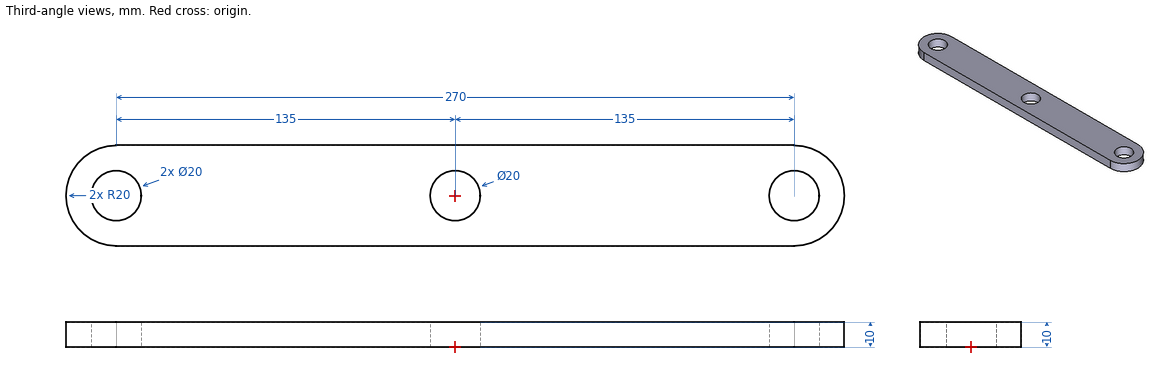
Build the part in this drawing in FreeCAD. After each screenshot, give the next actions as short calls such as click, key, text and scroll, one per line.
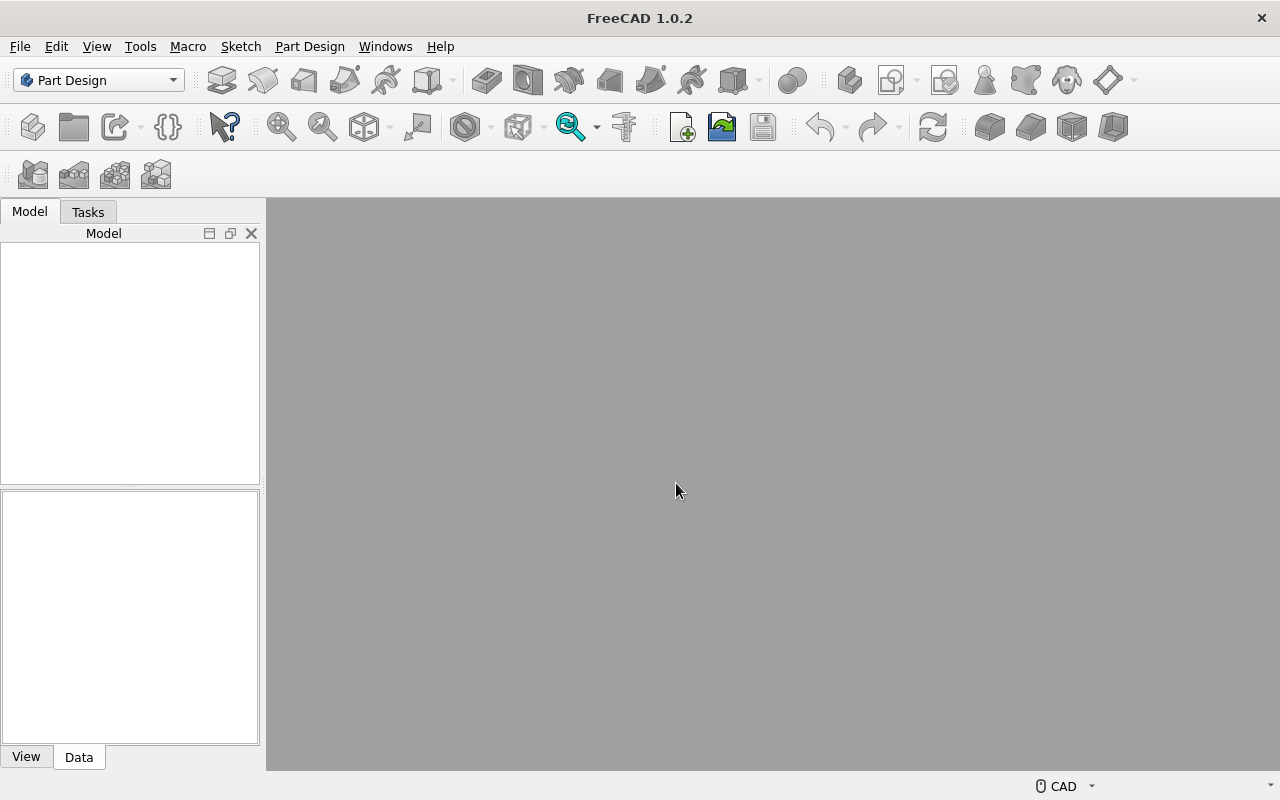
key(ctrl+n)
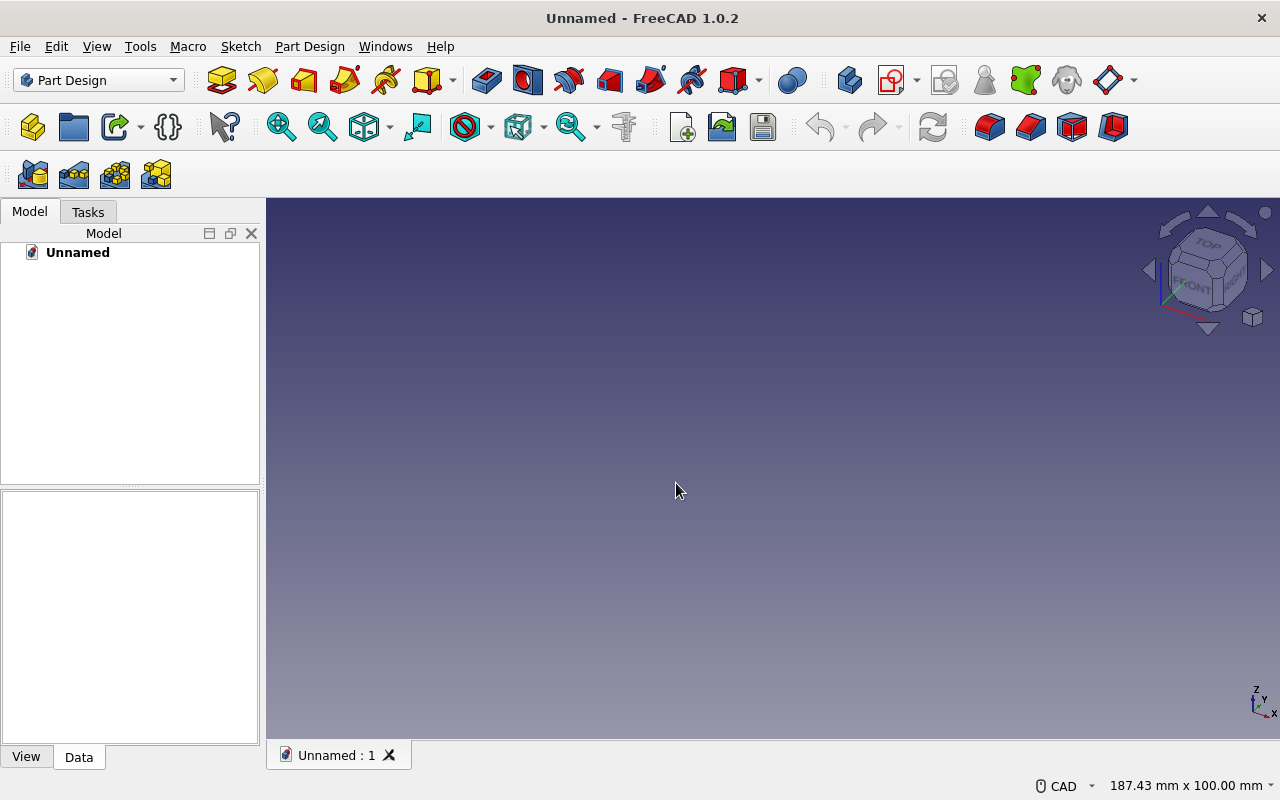
click(890, 80)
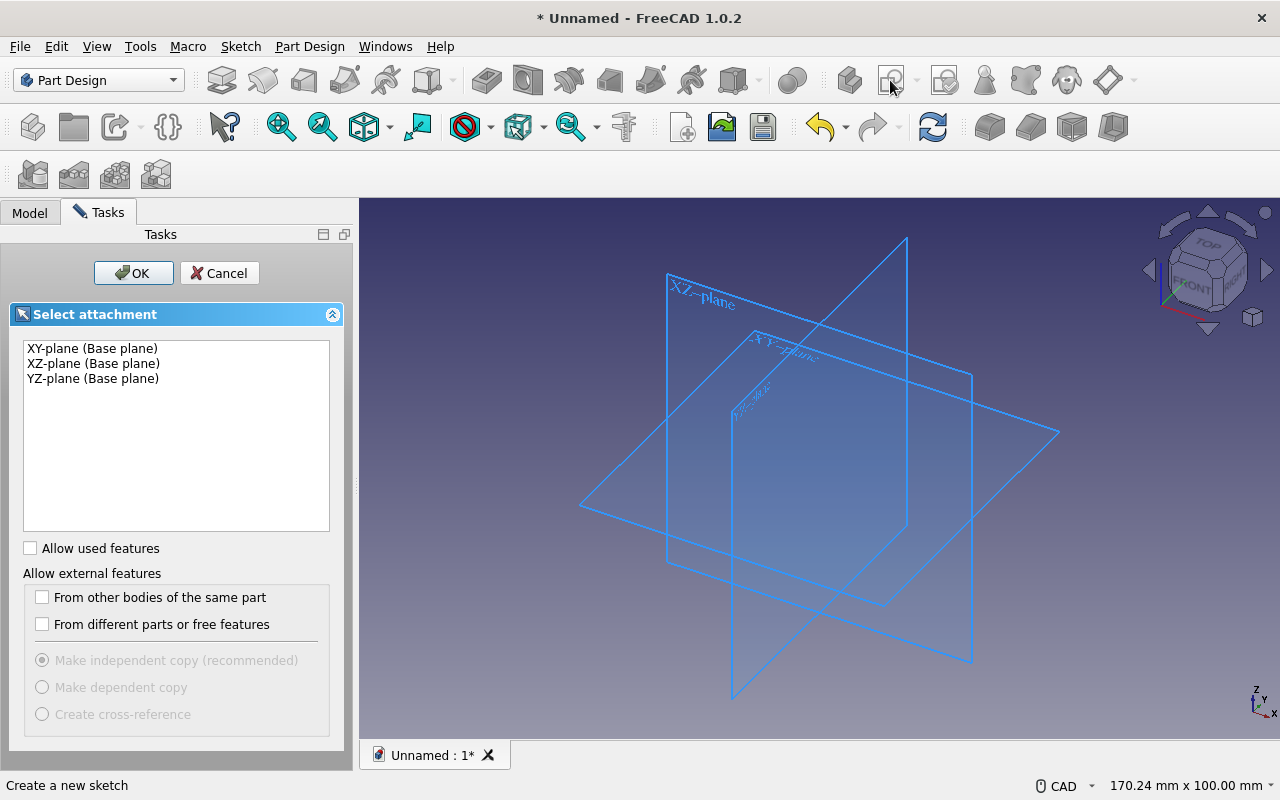
click(84, 348)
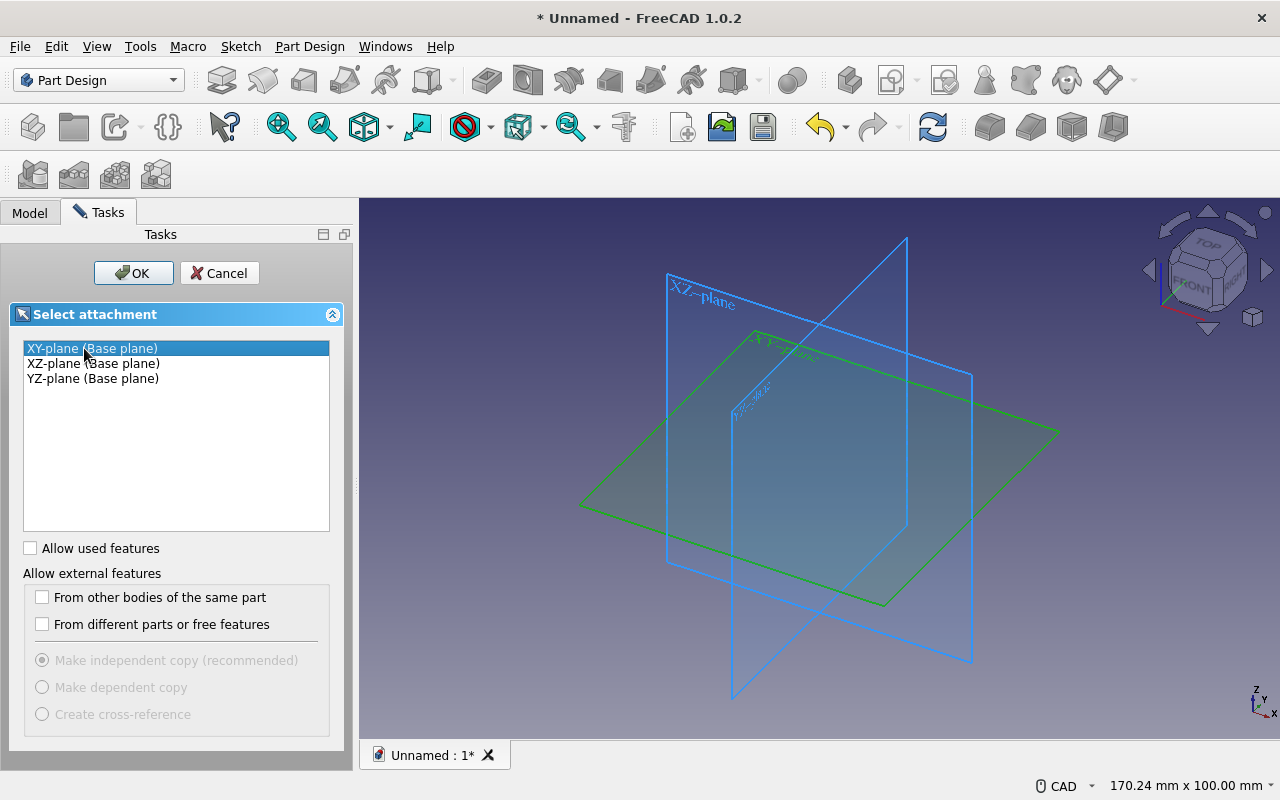
click(134, 273)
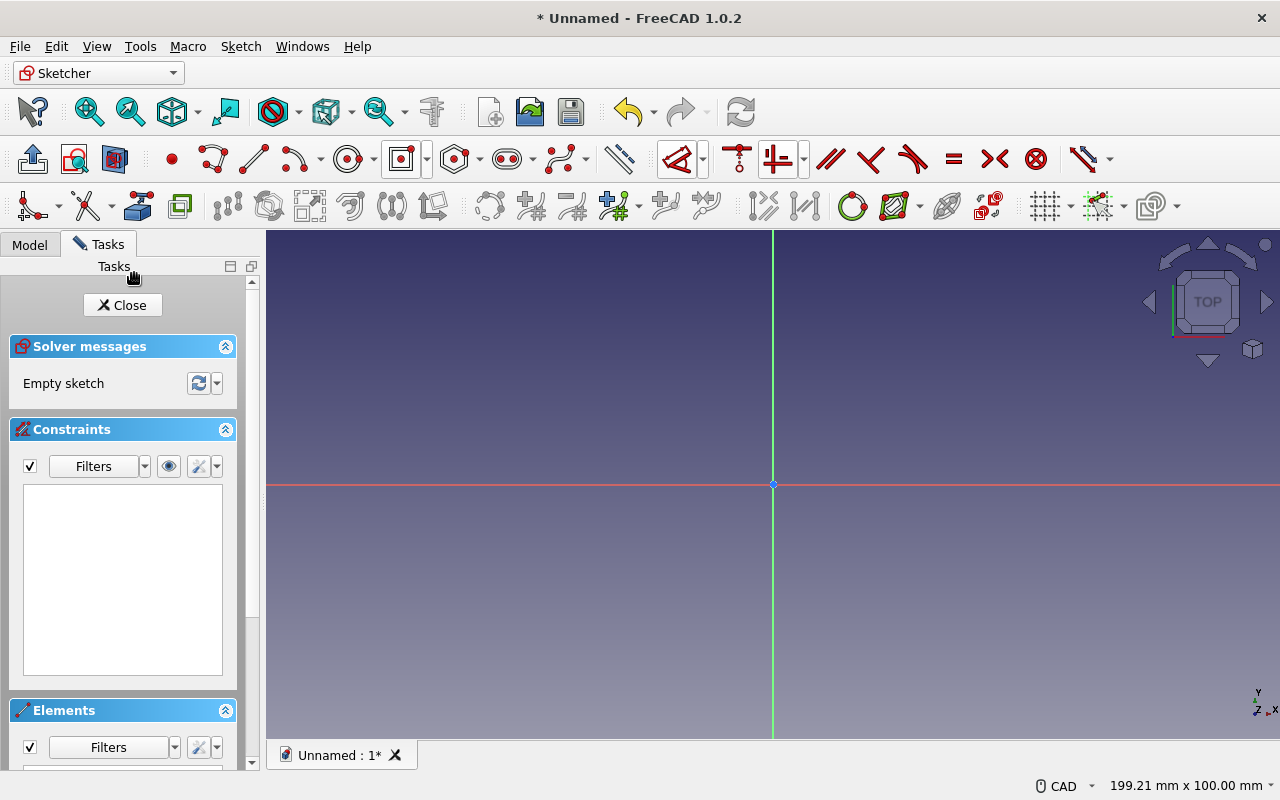
scroll(665, 484, down, 5)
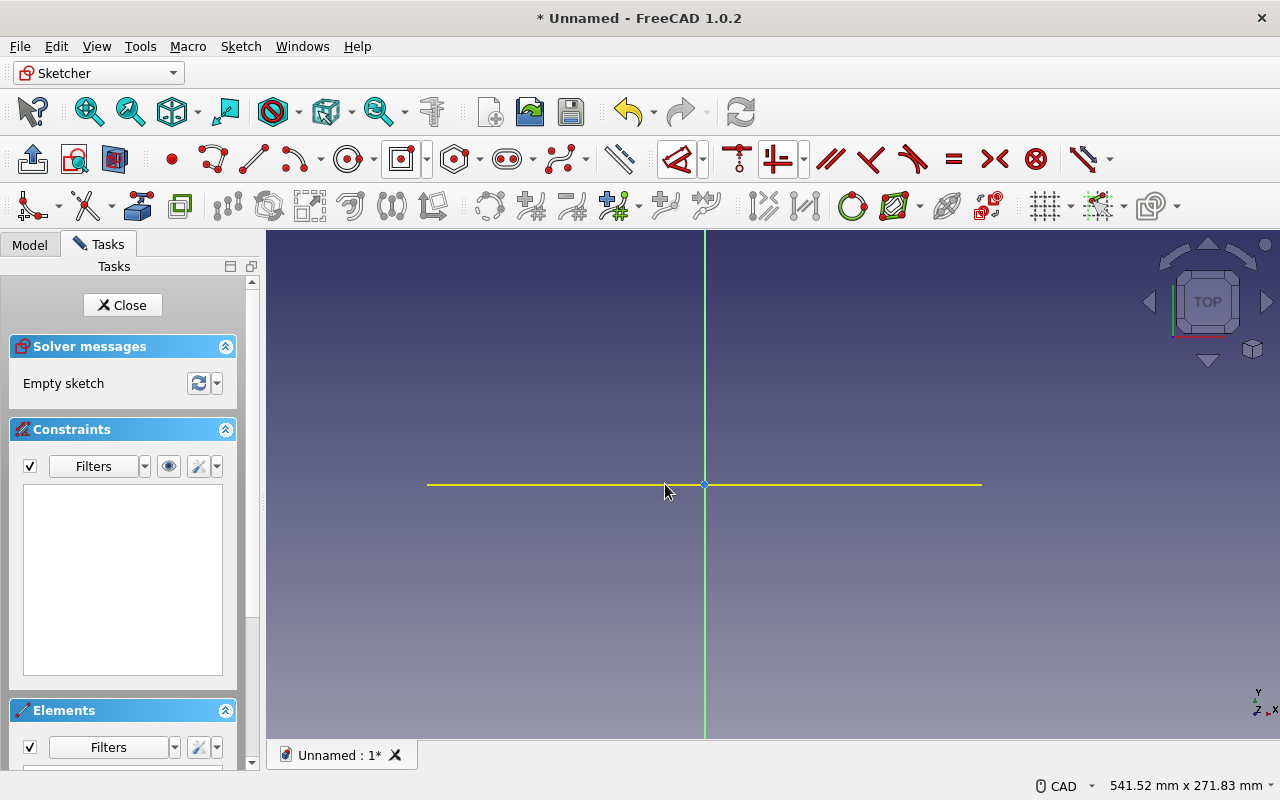
click(506, 160)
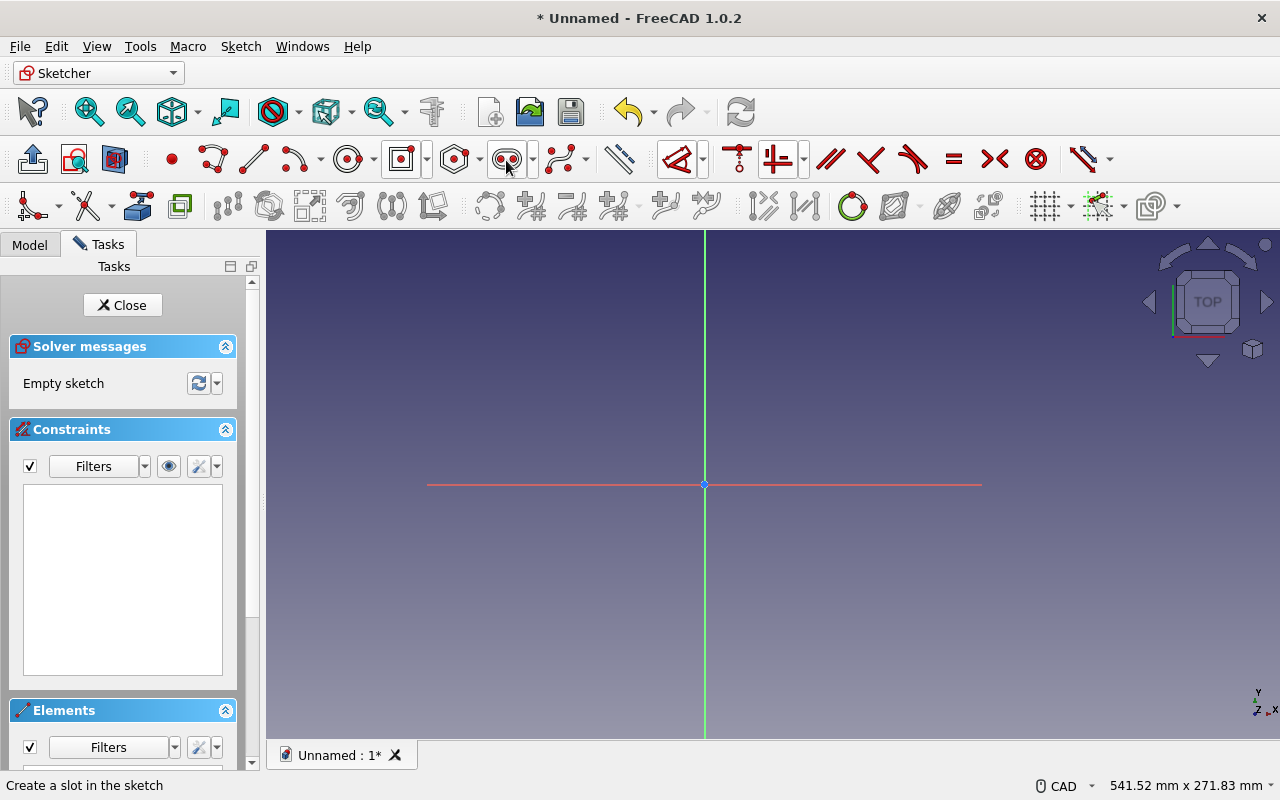
click(452, 484)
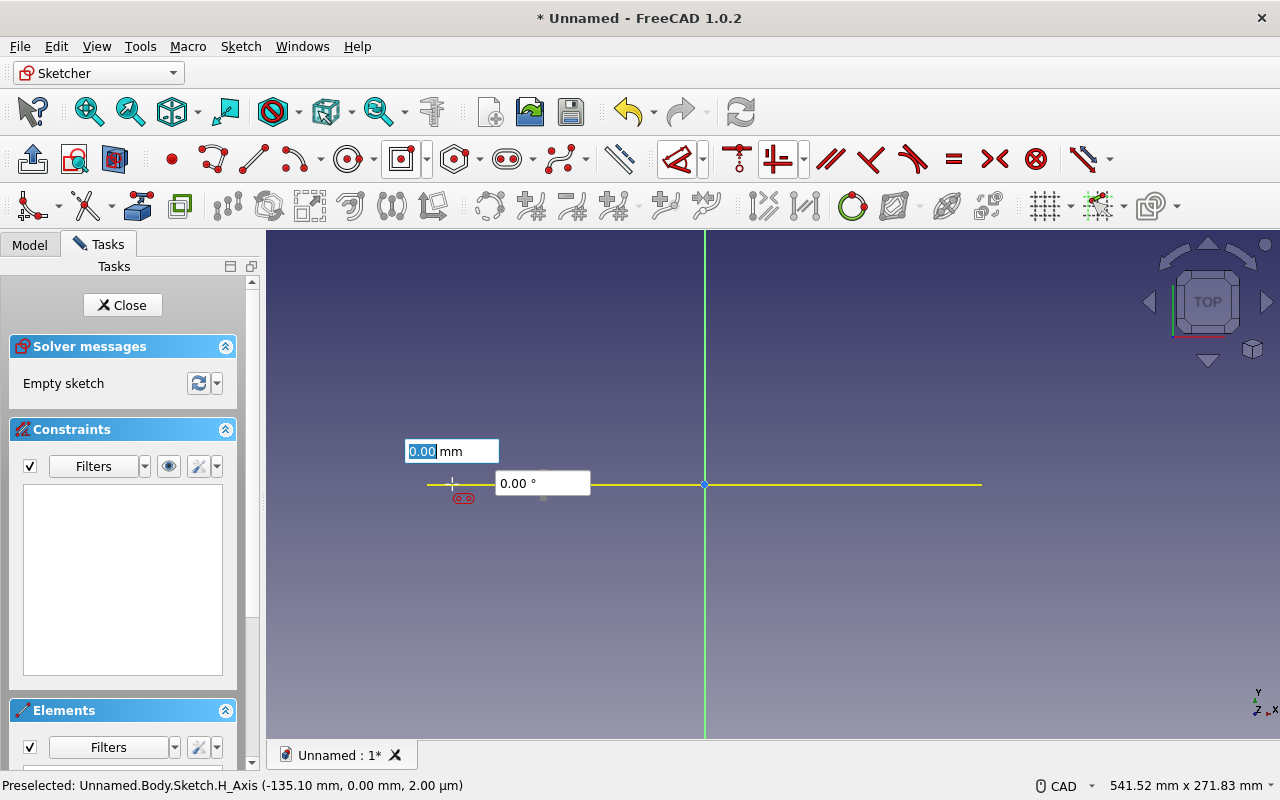
click(958, 476)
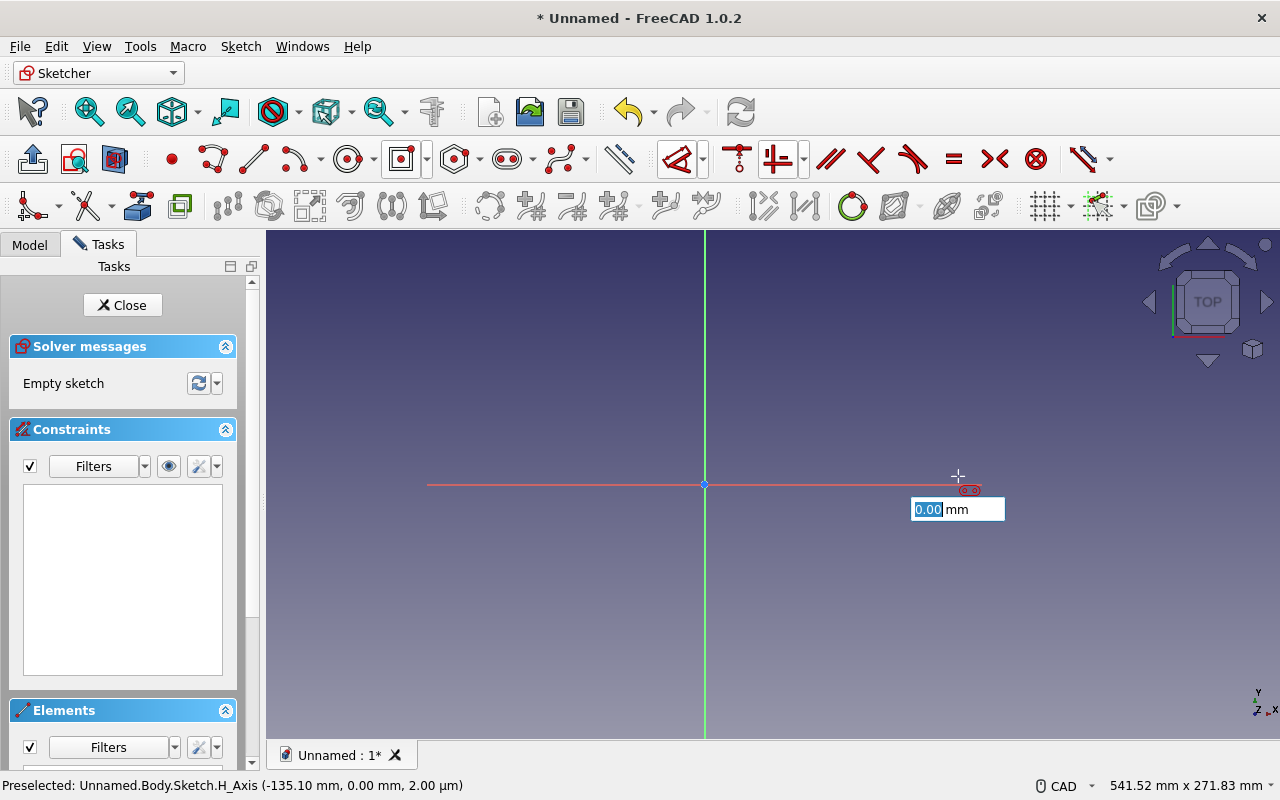
click(781, 447)
key(Escape)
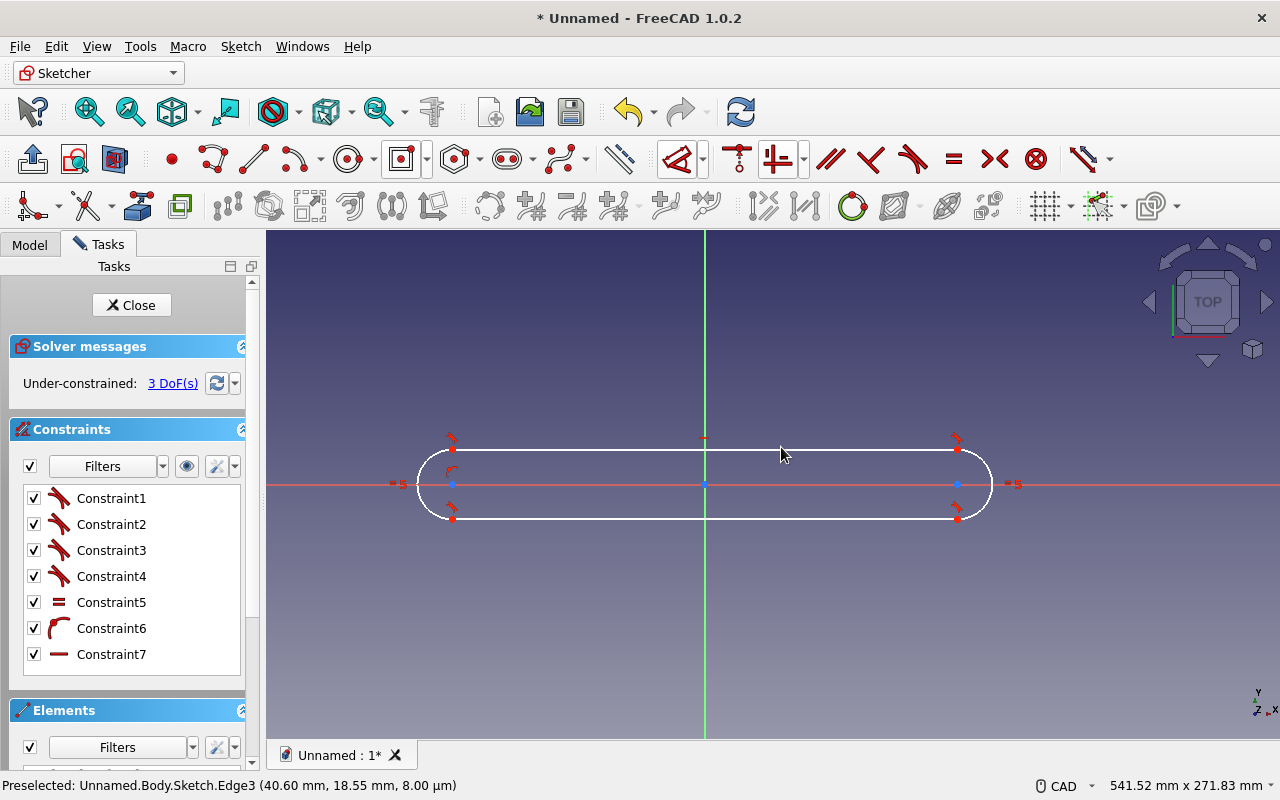
click(424, 464)